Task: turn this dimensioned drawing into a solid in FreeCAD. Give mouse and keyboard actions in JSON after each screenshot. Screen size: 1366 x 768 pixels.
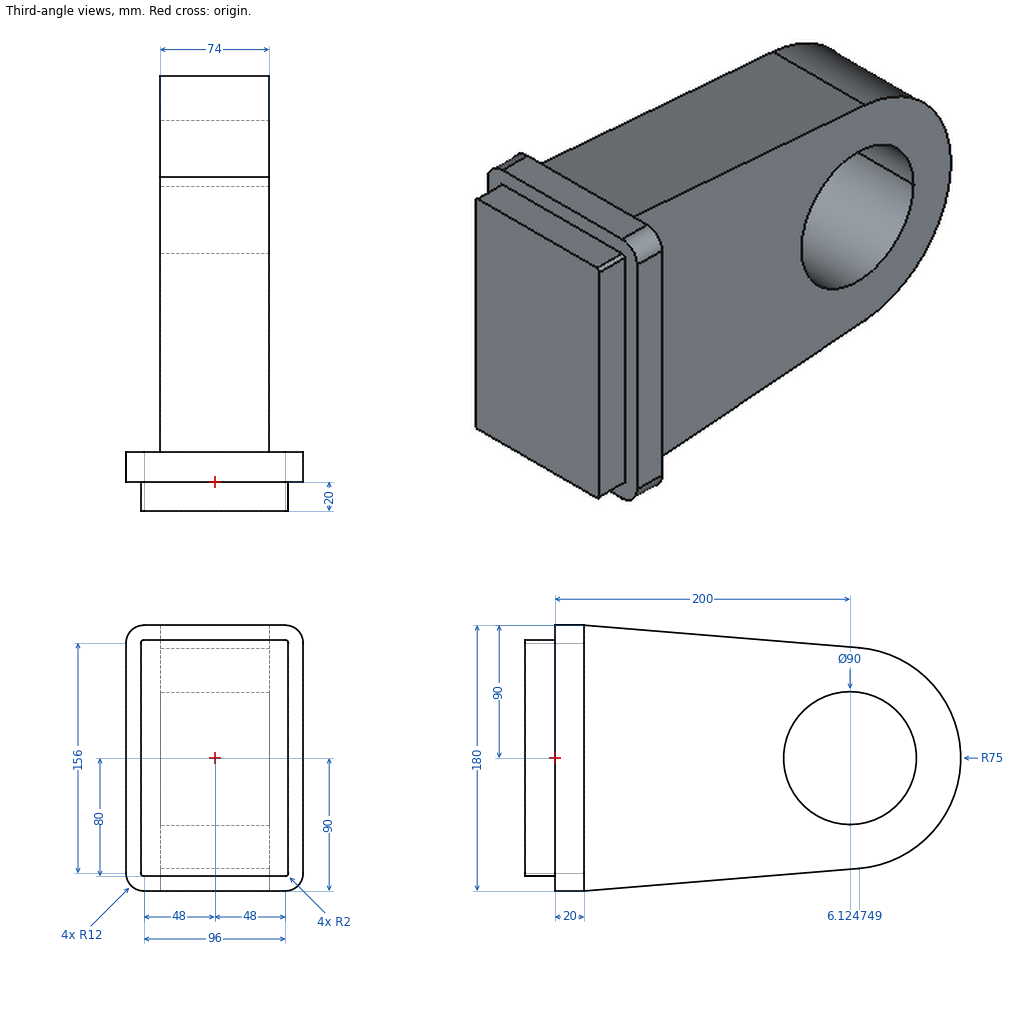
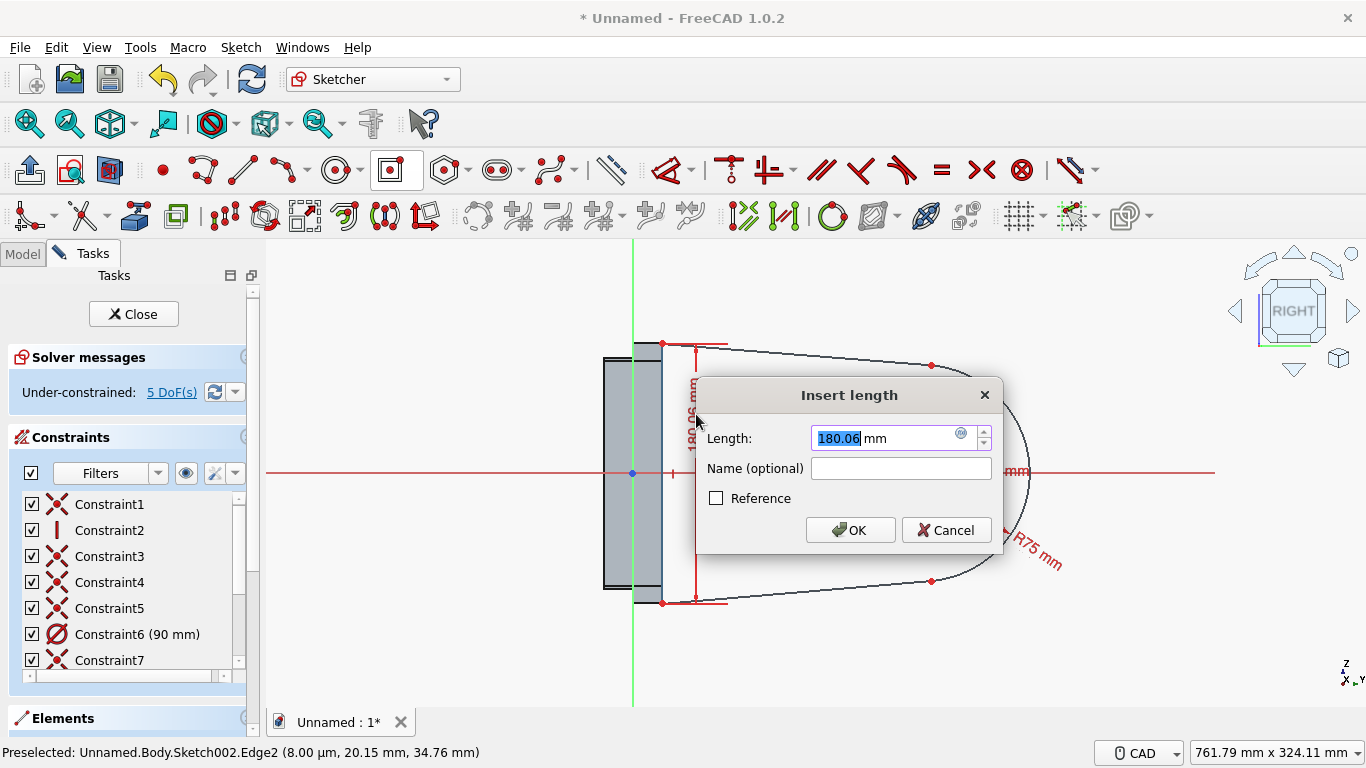
{"action": "type", "text": "180"}
{"action": "key", "text": "Return"}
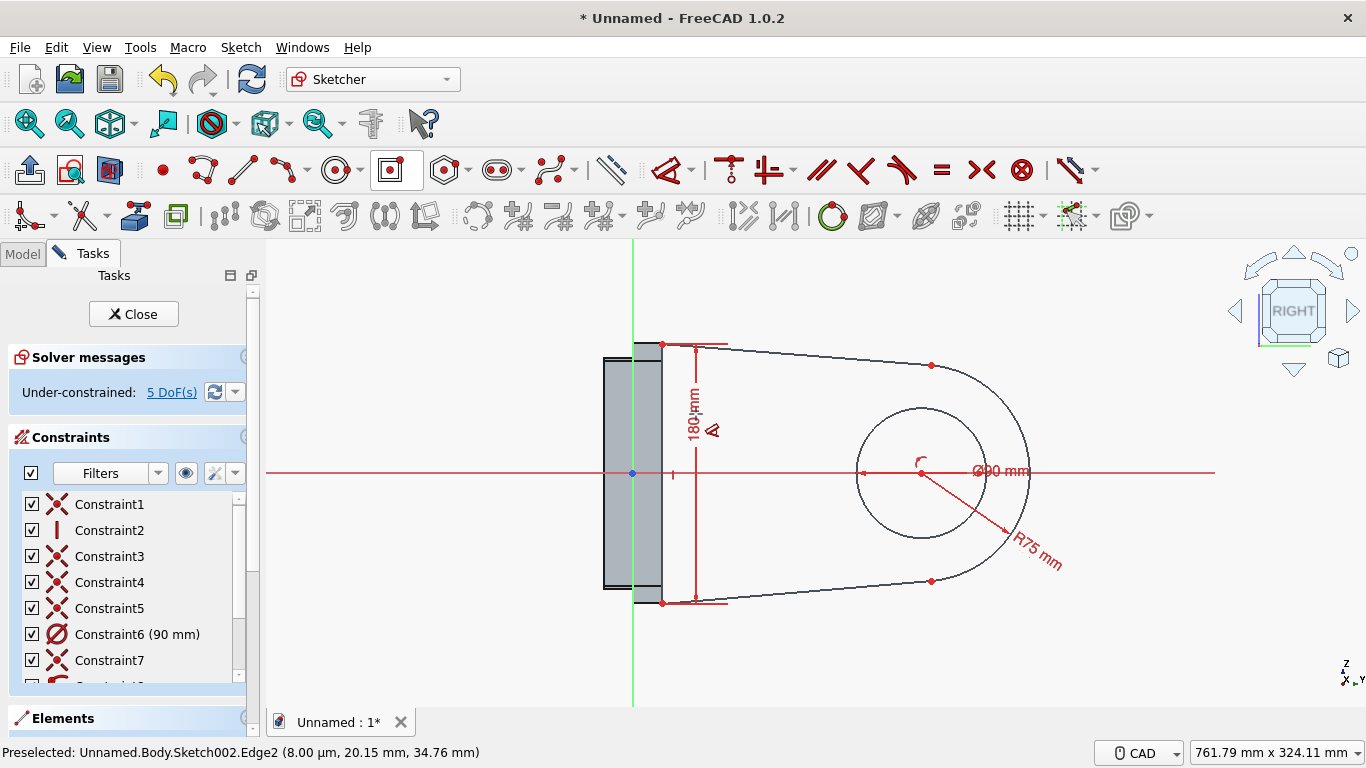
{"action": "scroll", "coordinate": [662, 344], "scroll_direction": "up", "scroll_amount": 2}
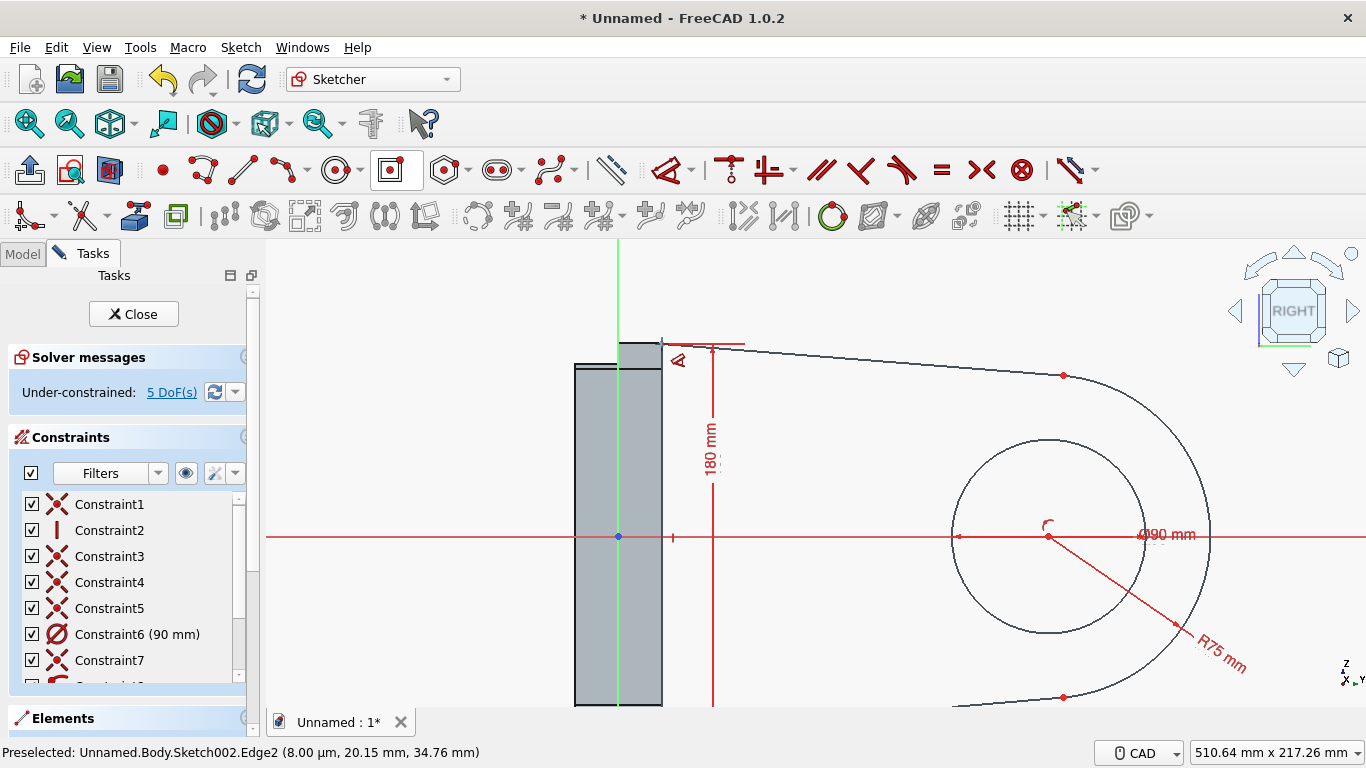
{"action": "left_click", "coordinate": [662, 344]}
{"action": "left_click", "coordinate": [640, 310]}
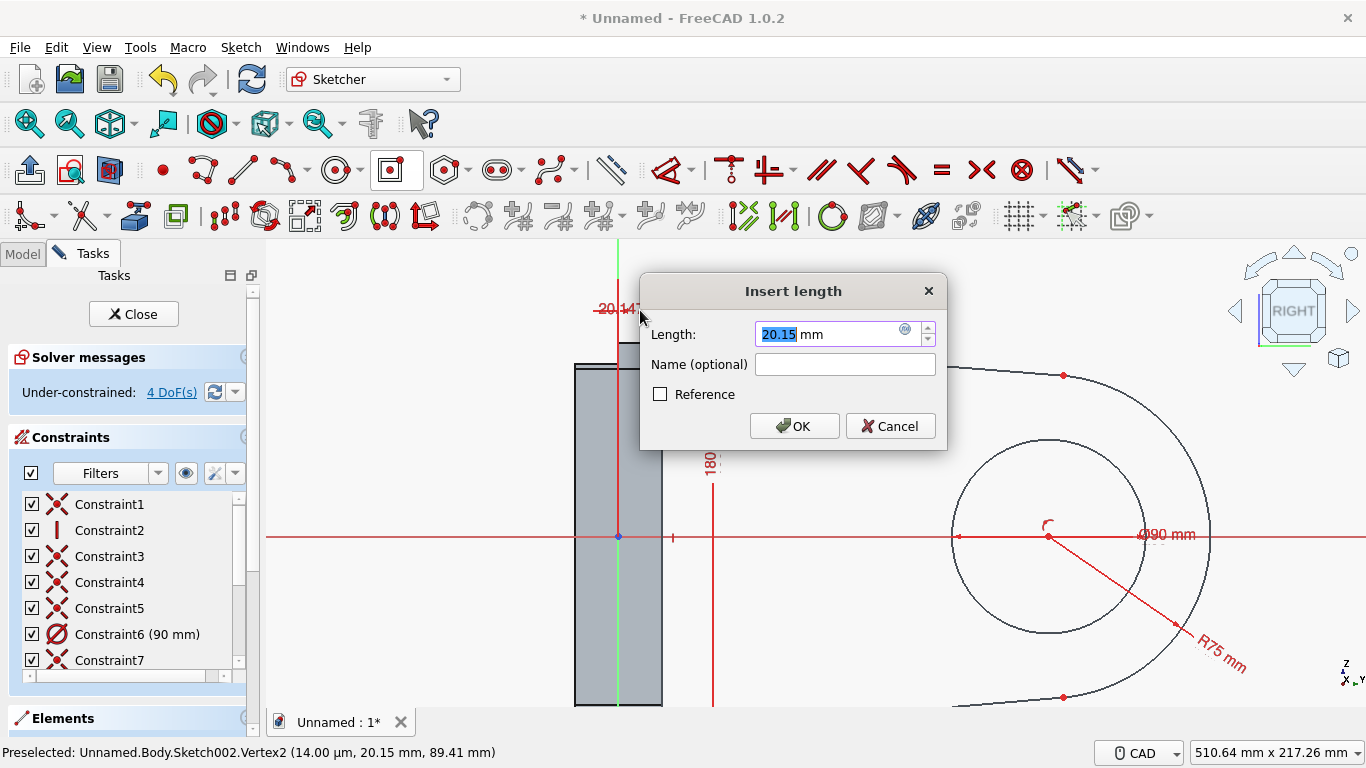
{"action": "type", "text": "20"}
{"action": "key", "text": "Return"}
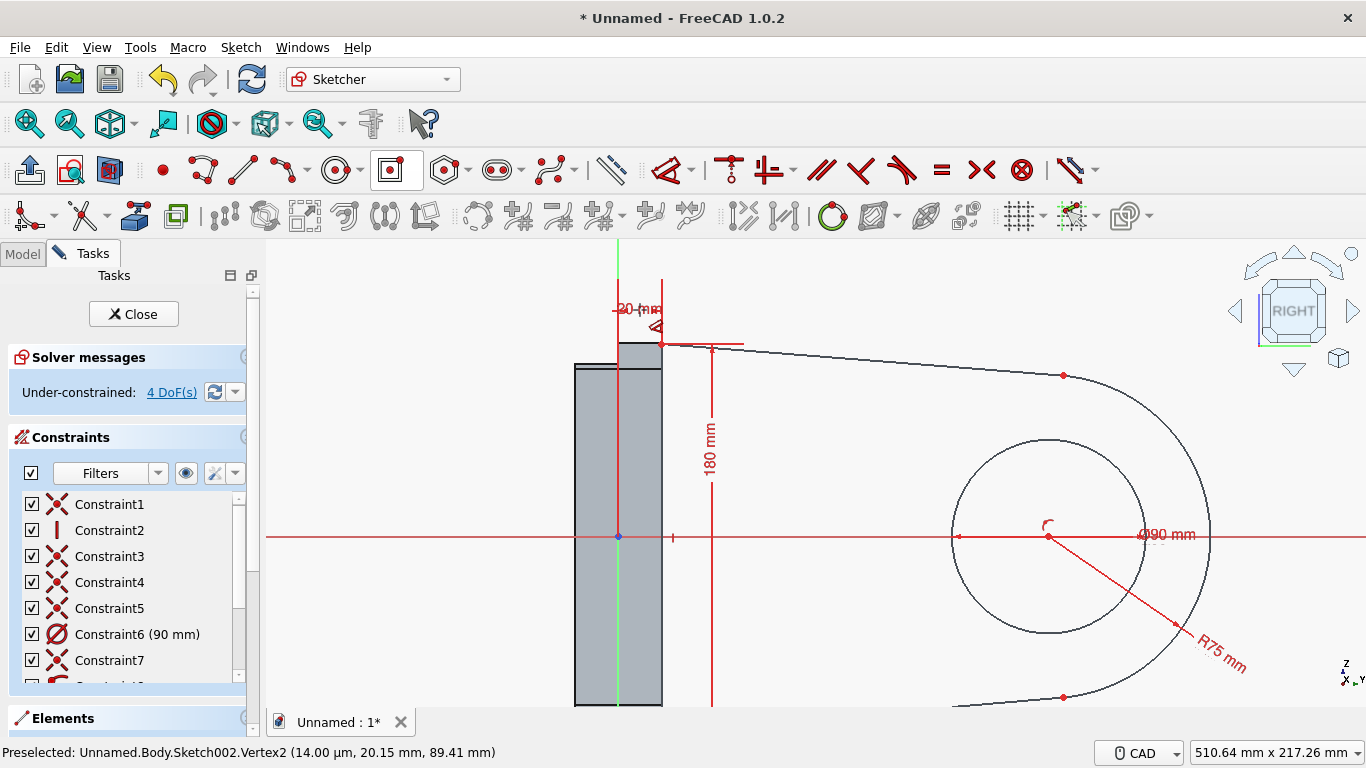
{"action": "left_click", "coordinate": [662, 344]}
{"action": "left_click", "coordinate": [584, 440]}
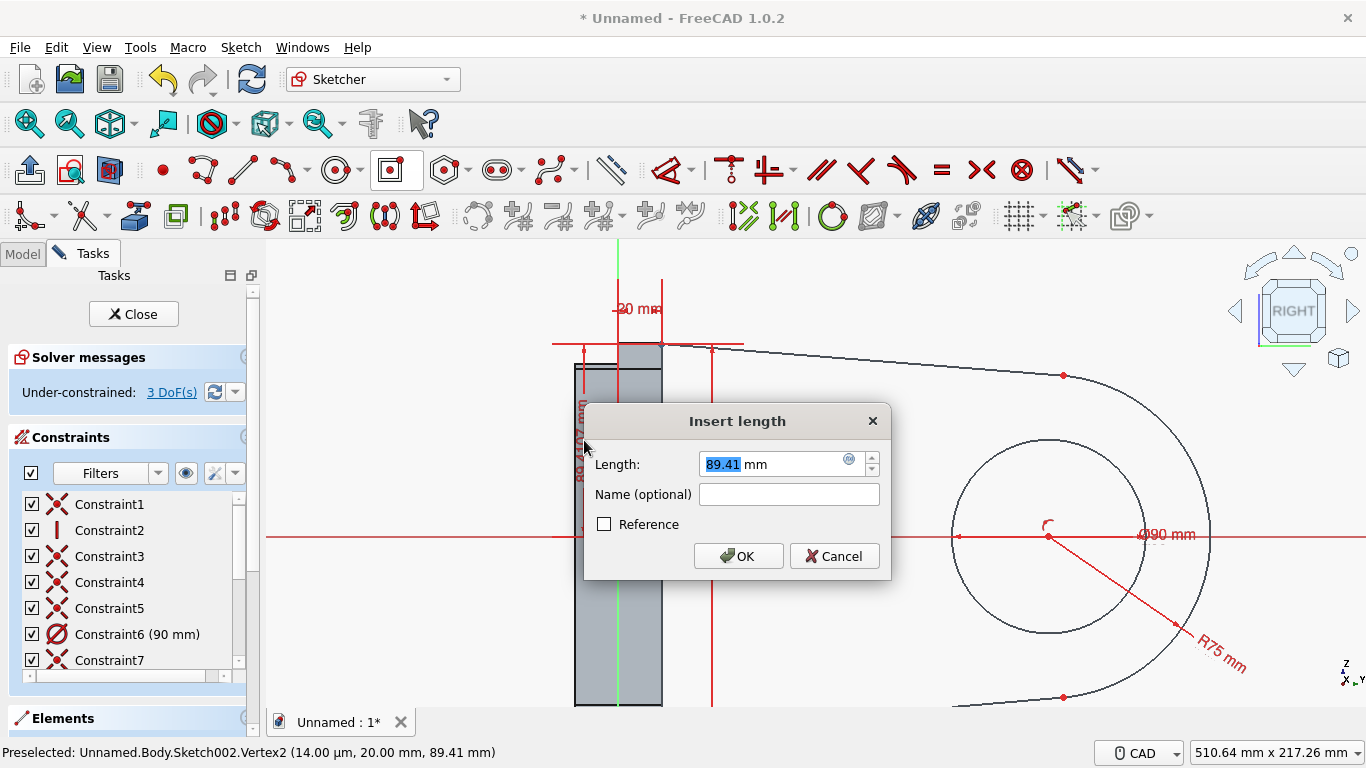
{"action": "type", "text": "90"}
{"action": "key", "text": "Return"}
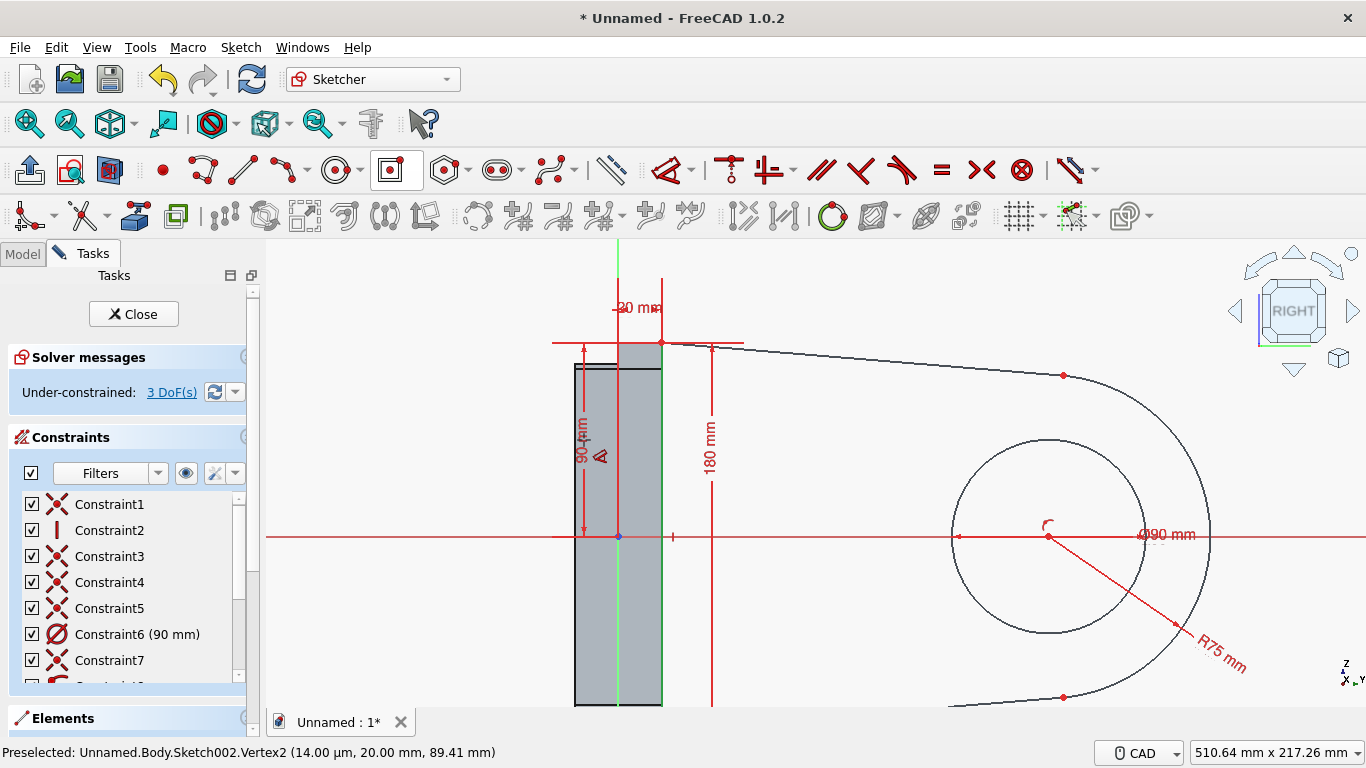
{"action": "left_click", "coordinate": [1049, 537]}
{"action": "left_click", "coordinate": [834, 571]}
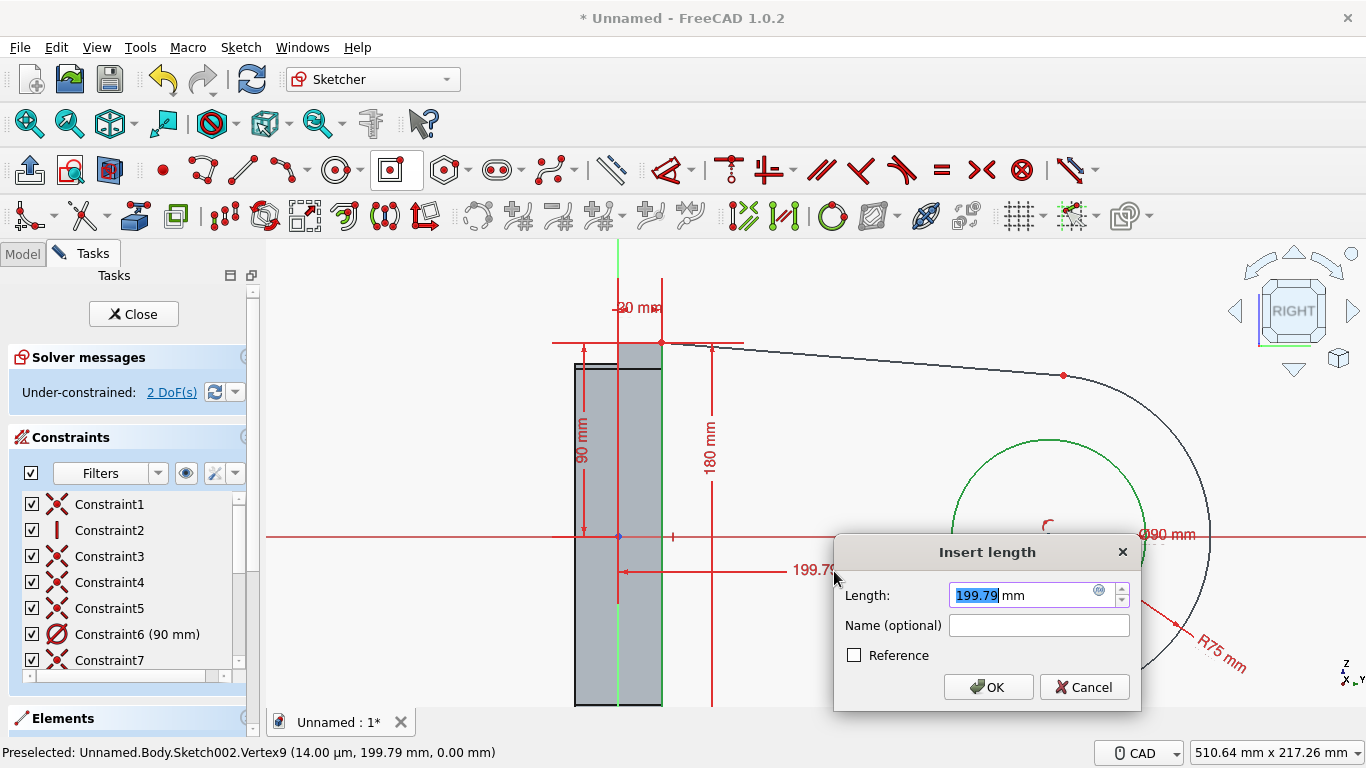
{"action": "type", "text": "200"}
{"action": "key", "text": "Return"}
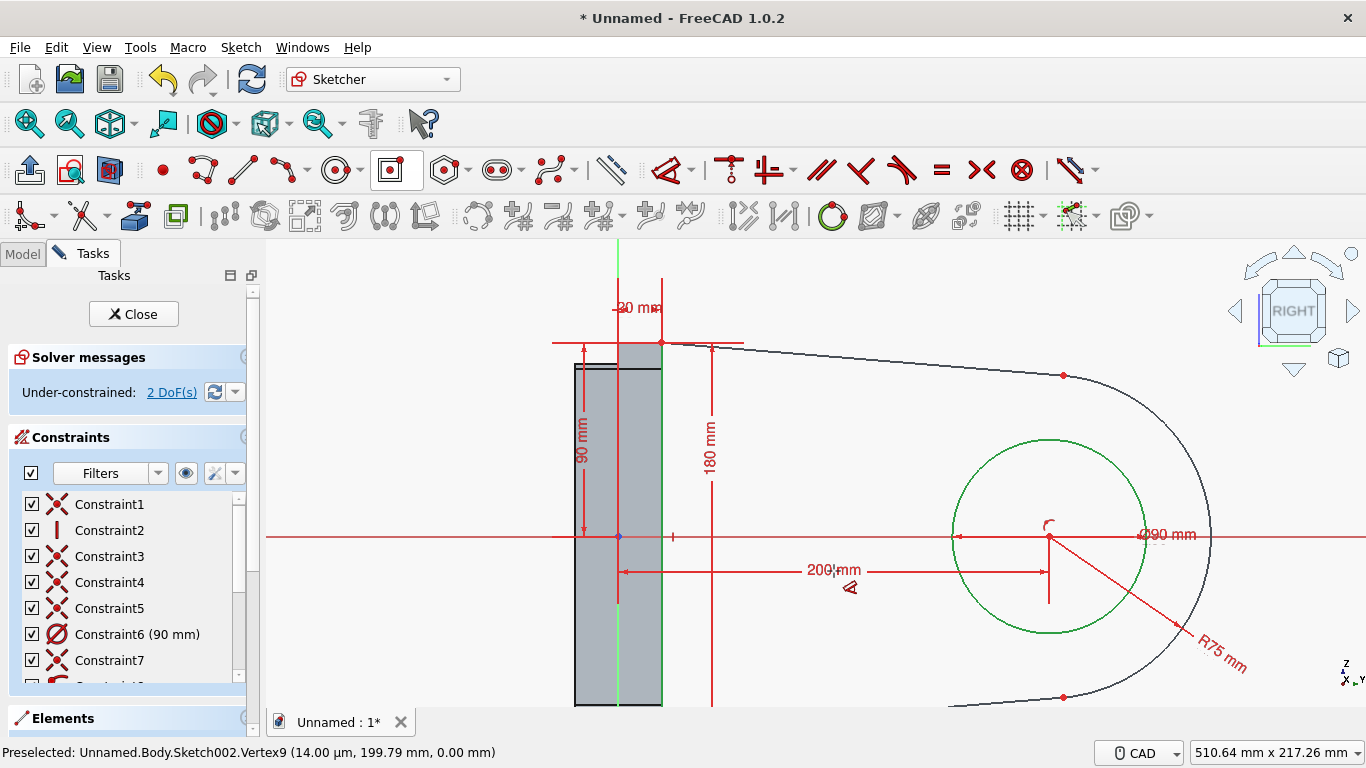
{"action": "scroll", "coordinate": [294, 267], "scroll_direction": "down", "scroll_amount": 1}